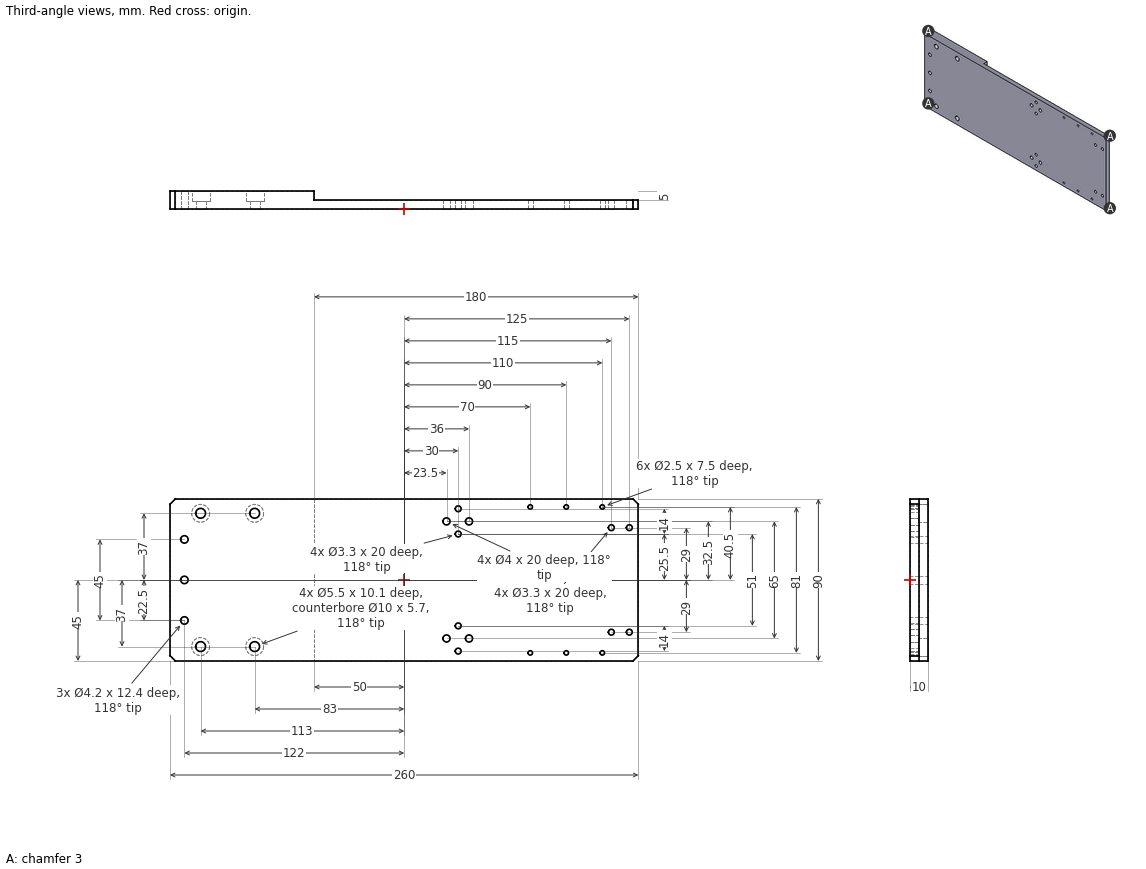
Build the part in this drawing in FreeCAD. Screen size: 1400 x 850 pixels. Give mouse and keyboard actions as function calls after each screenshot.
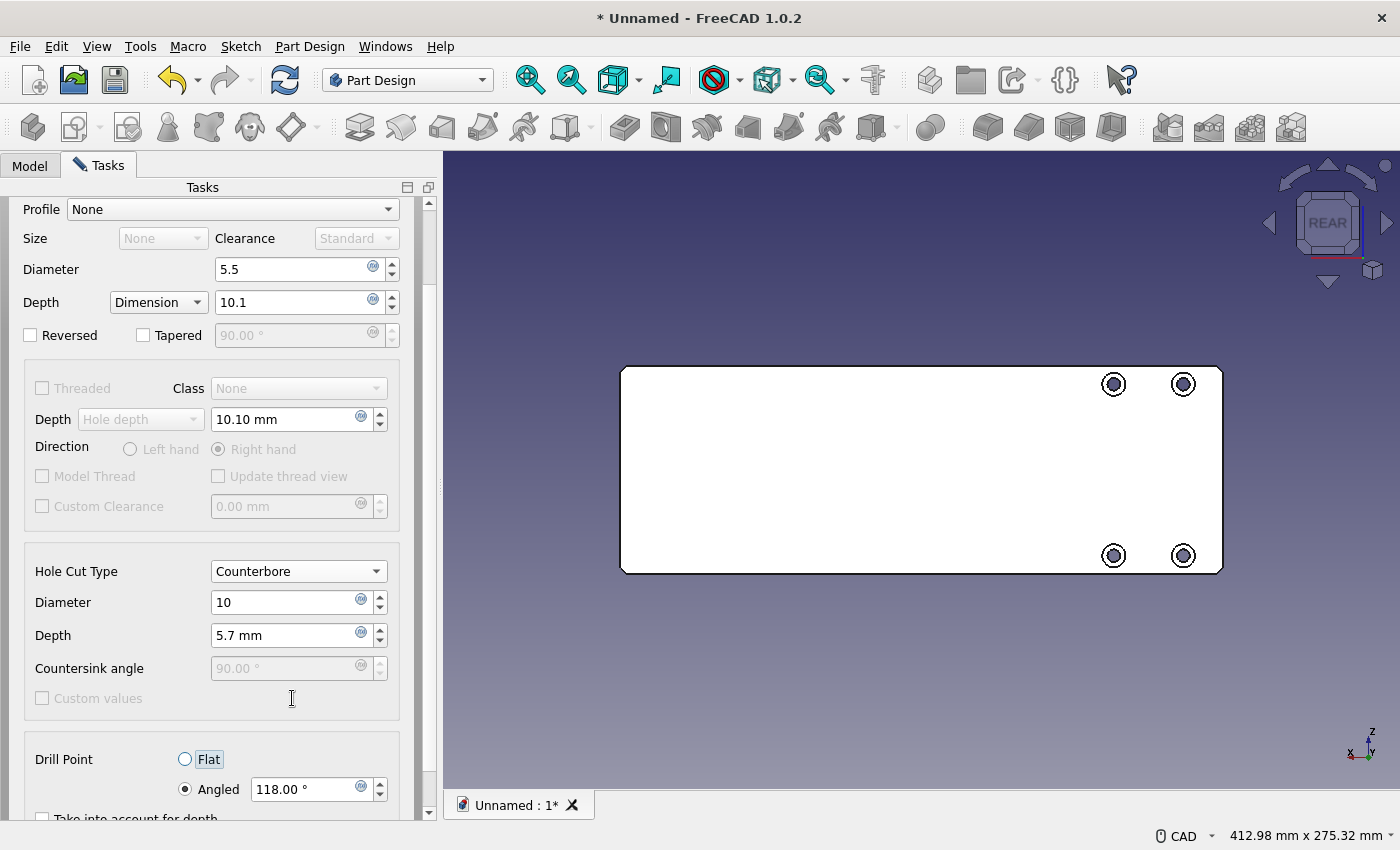
scroll(429, 508, up, 3)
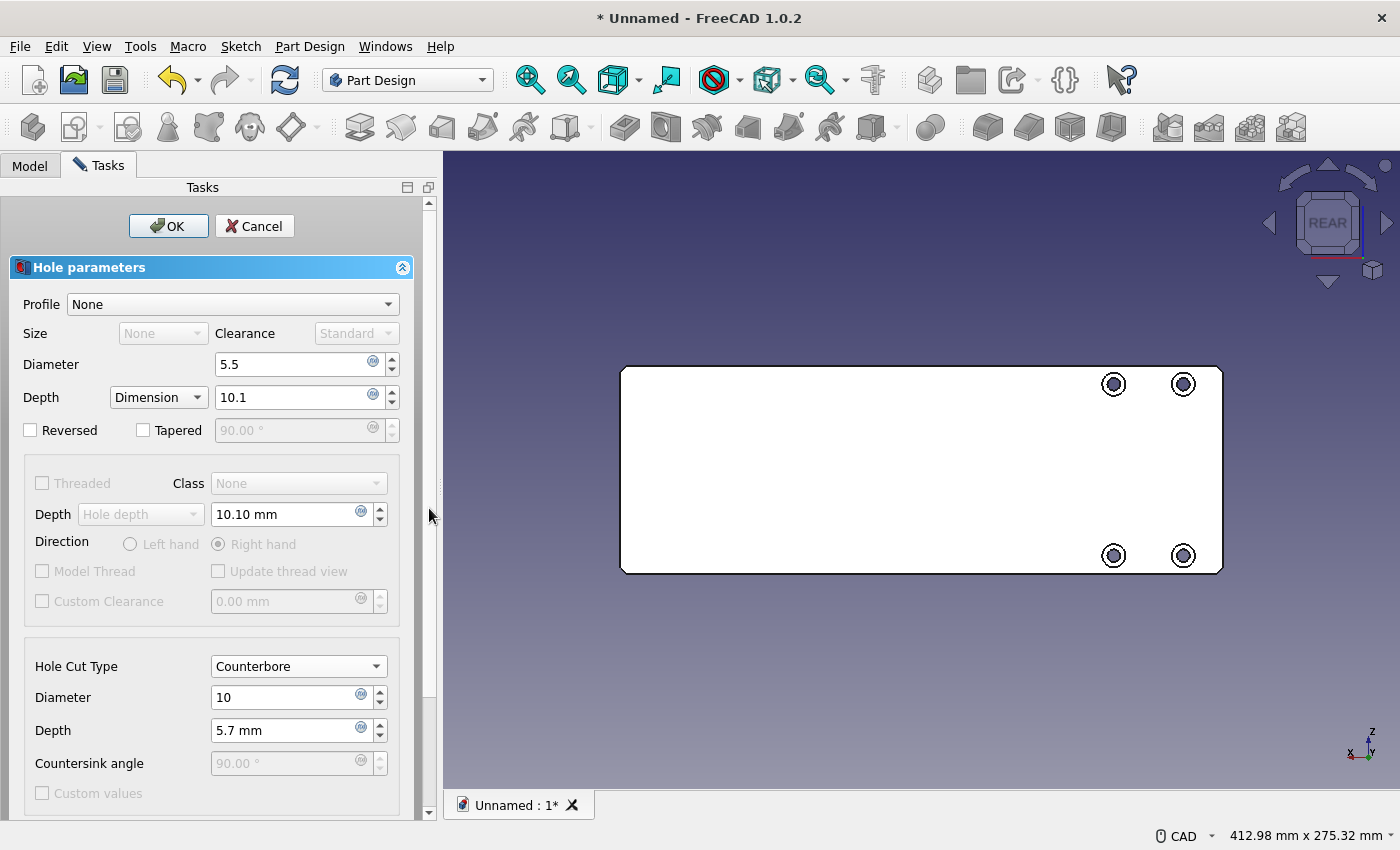
click(169, 226)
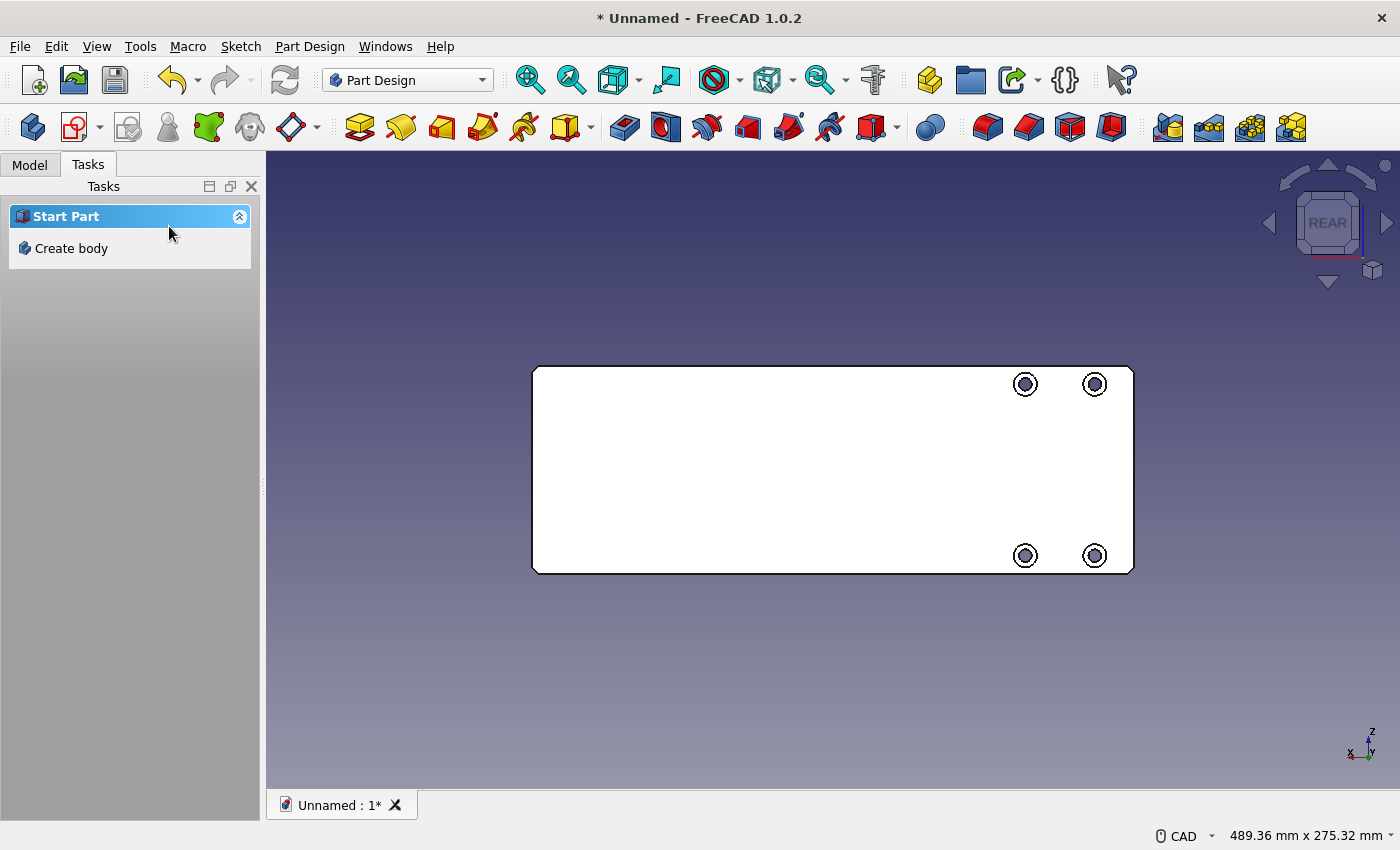
click(661, 469)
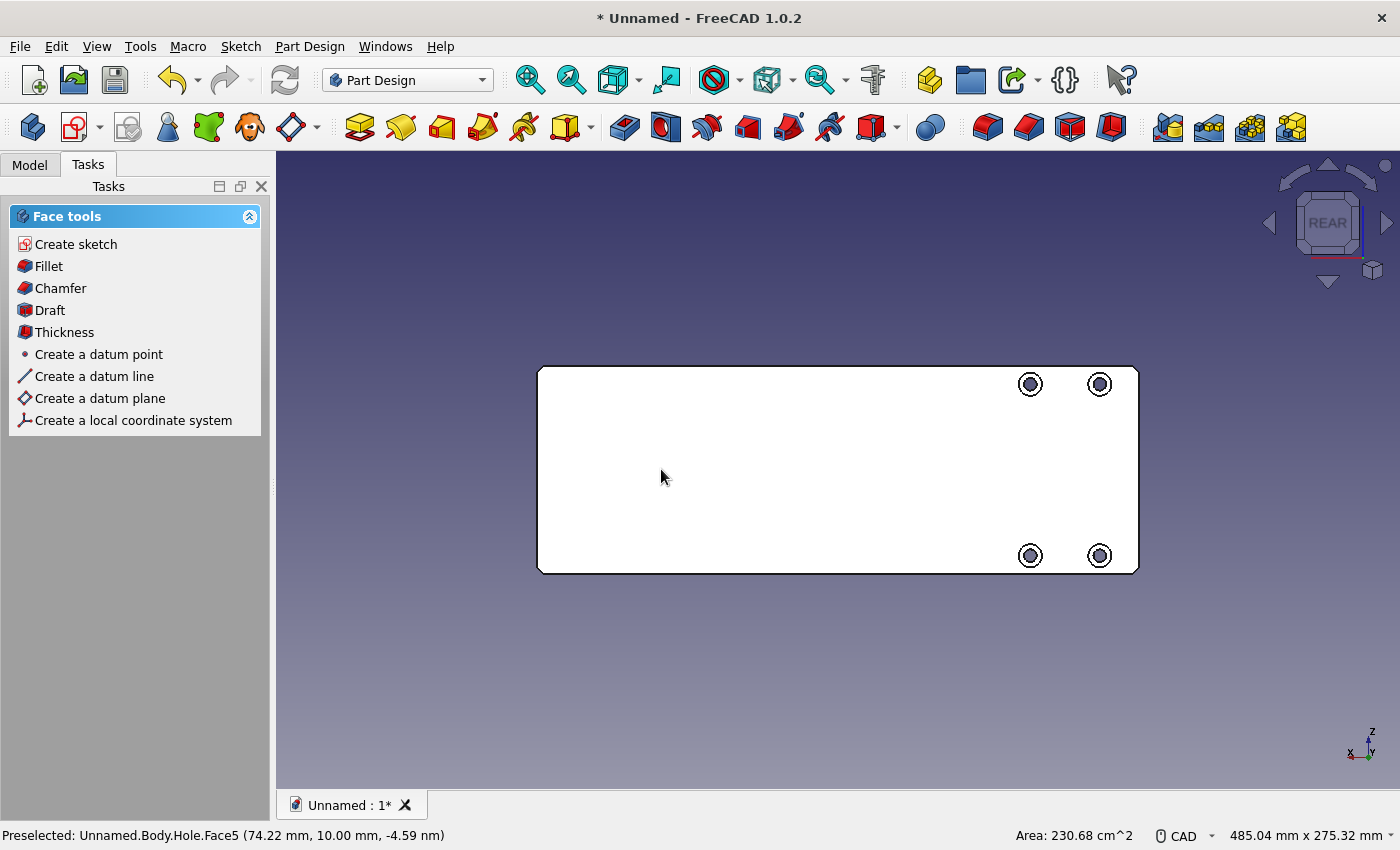
click(74, 128)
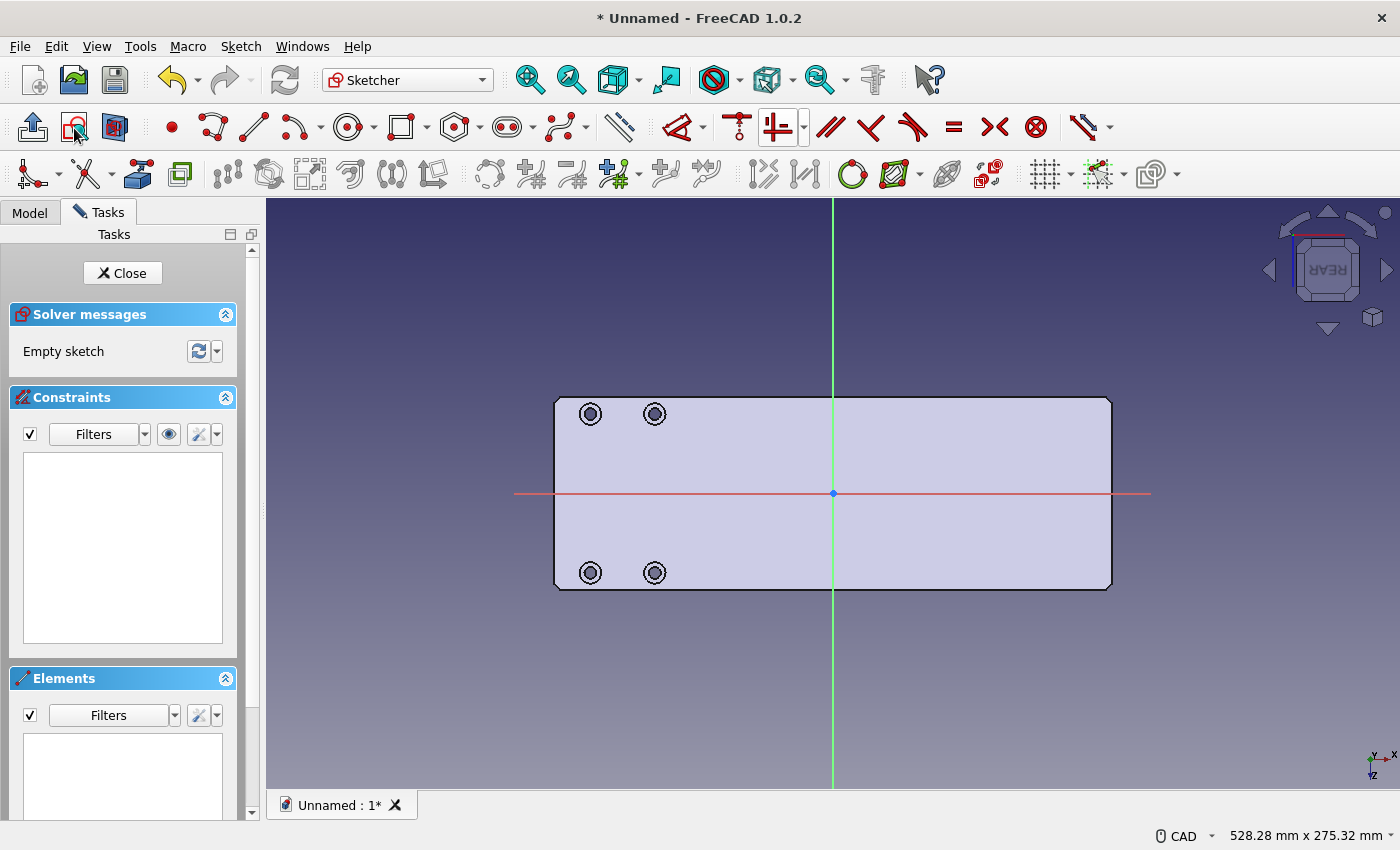
scroll(488, 493, up, 6)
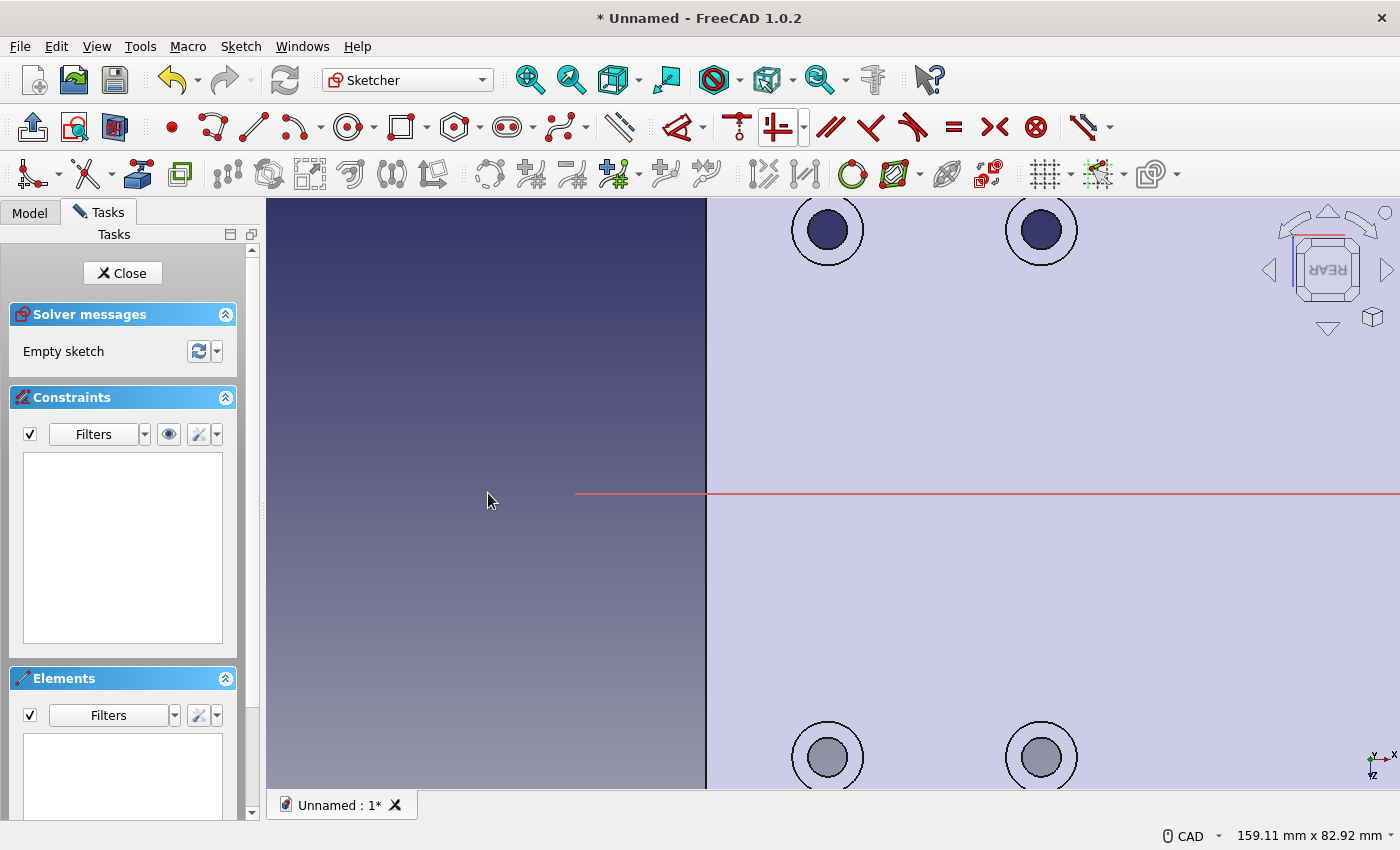
click(348, 128)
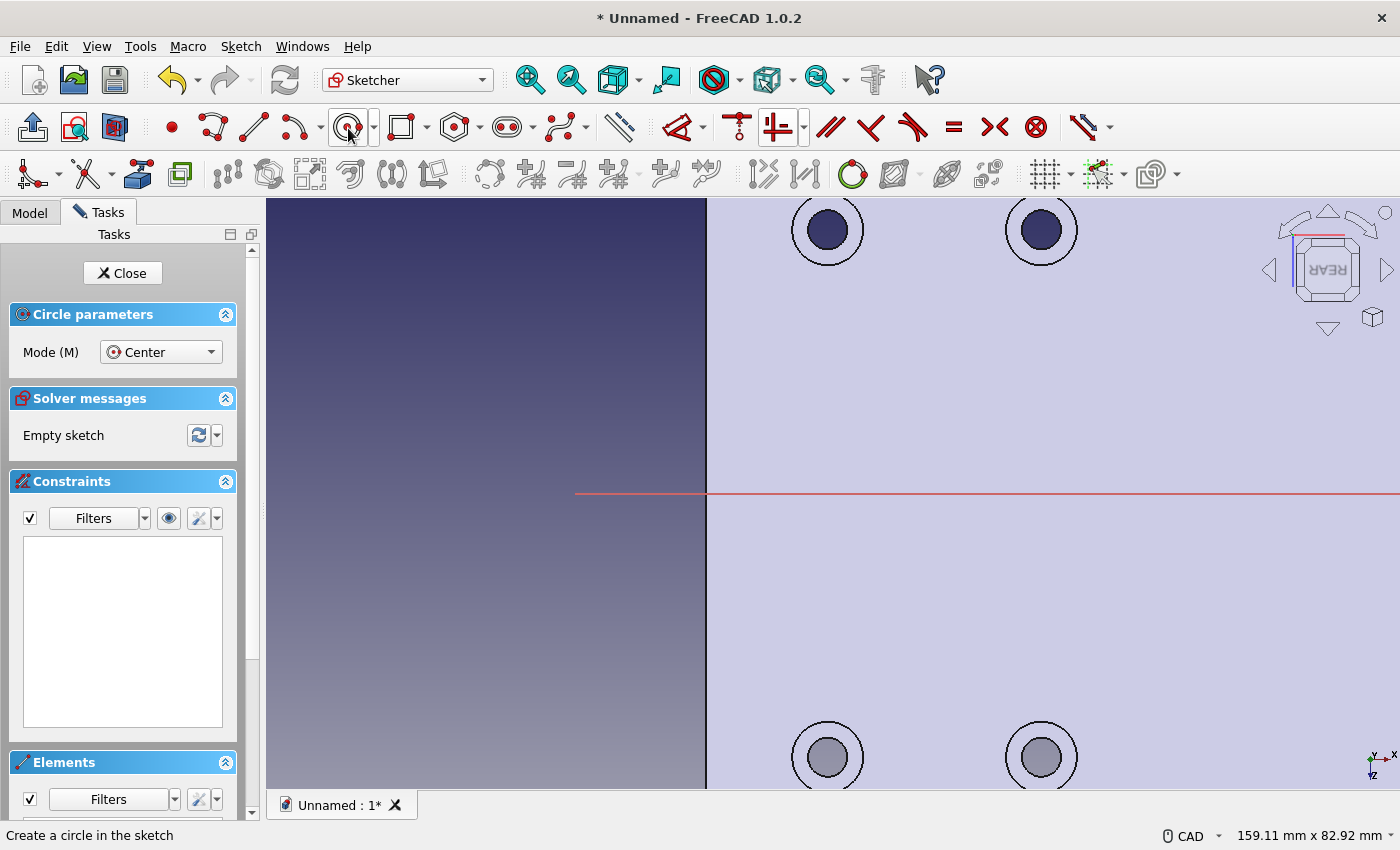
scroll(763, 333, up, 3)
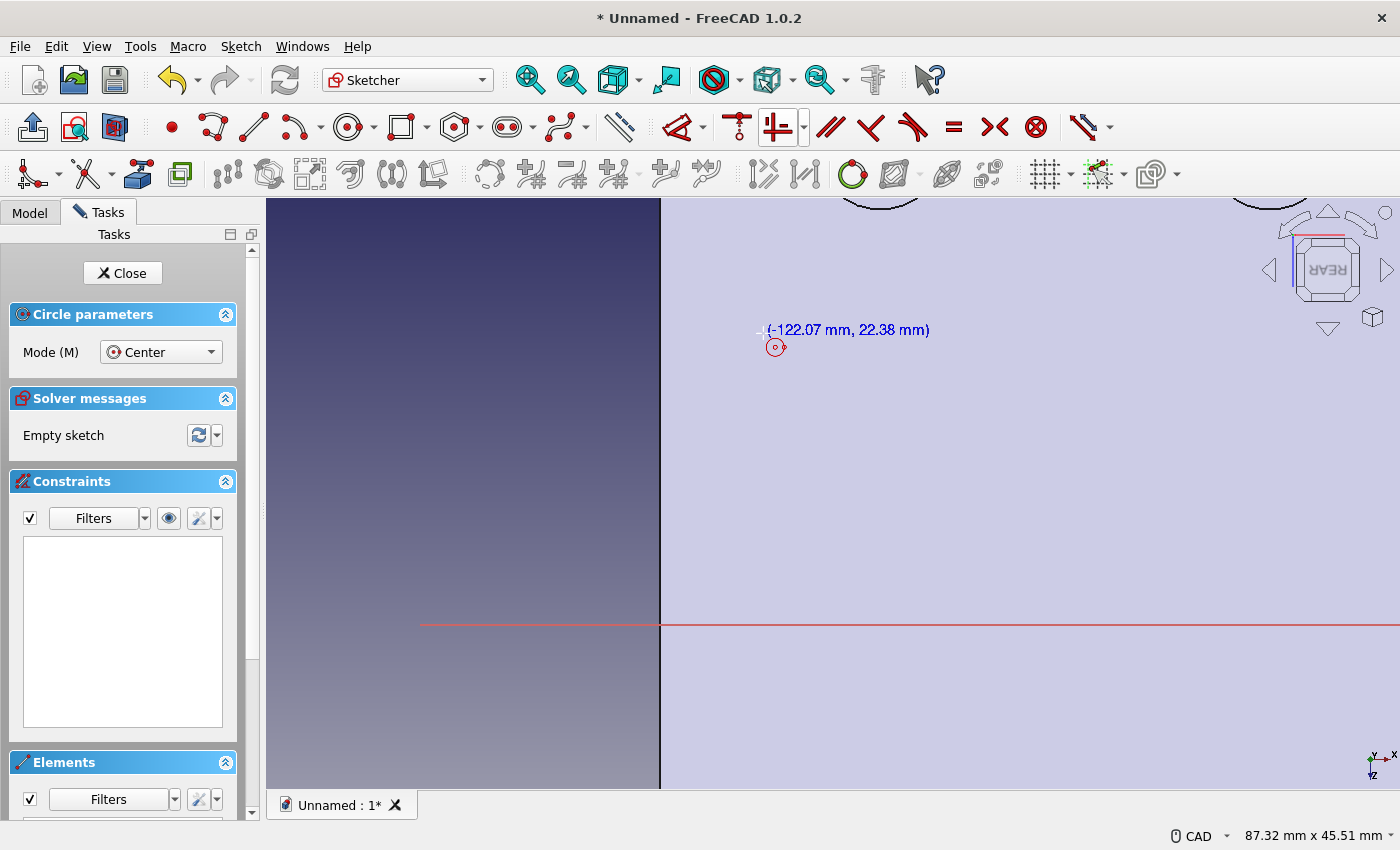
click(764, 333)
click(783, 314)